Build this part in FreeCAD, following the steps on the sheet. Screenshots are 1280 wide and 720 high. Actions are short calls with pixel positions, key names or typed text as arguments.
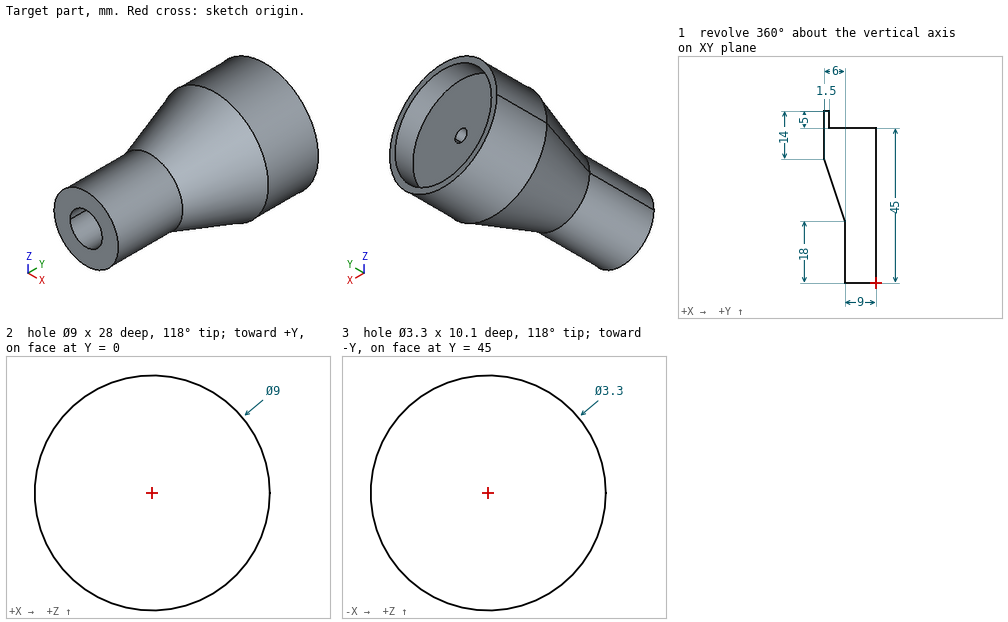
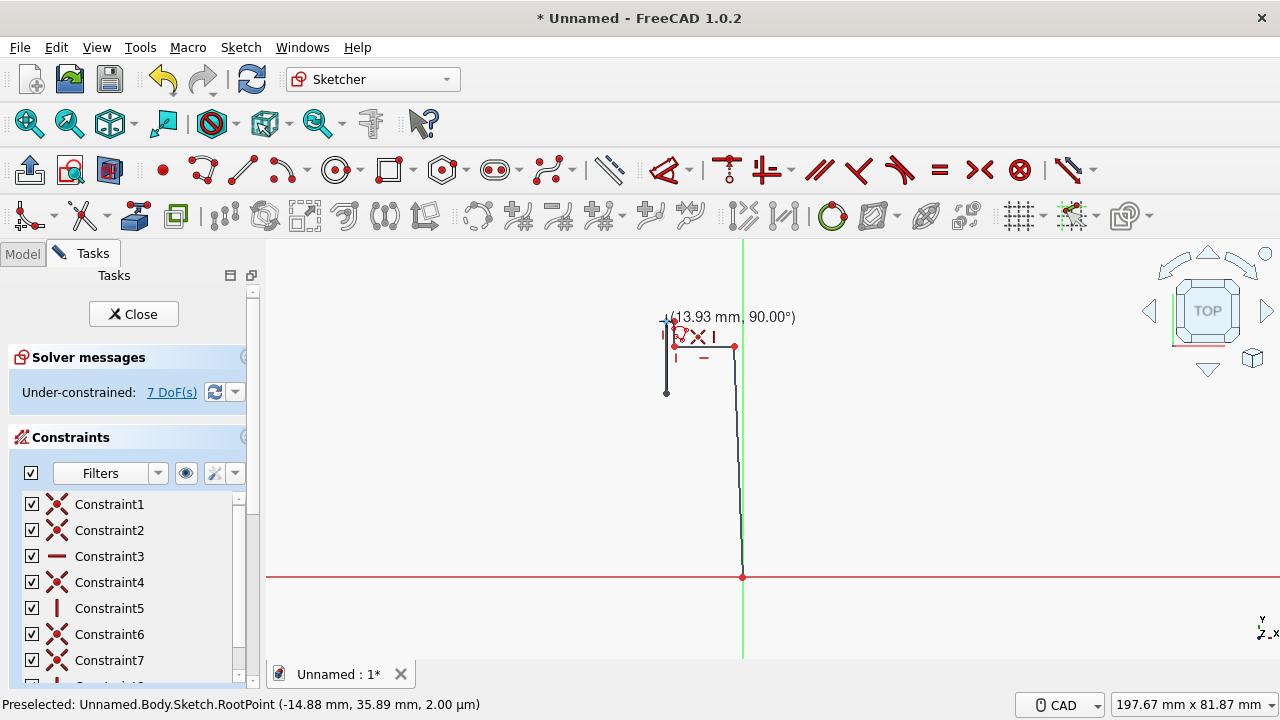
click(697, 485)
click(697, 568)
click(743, 577)
key(Escape)
key(Escape)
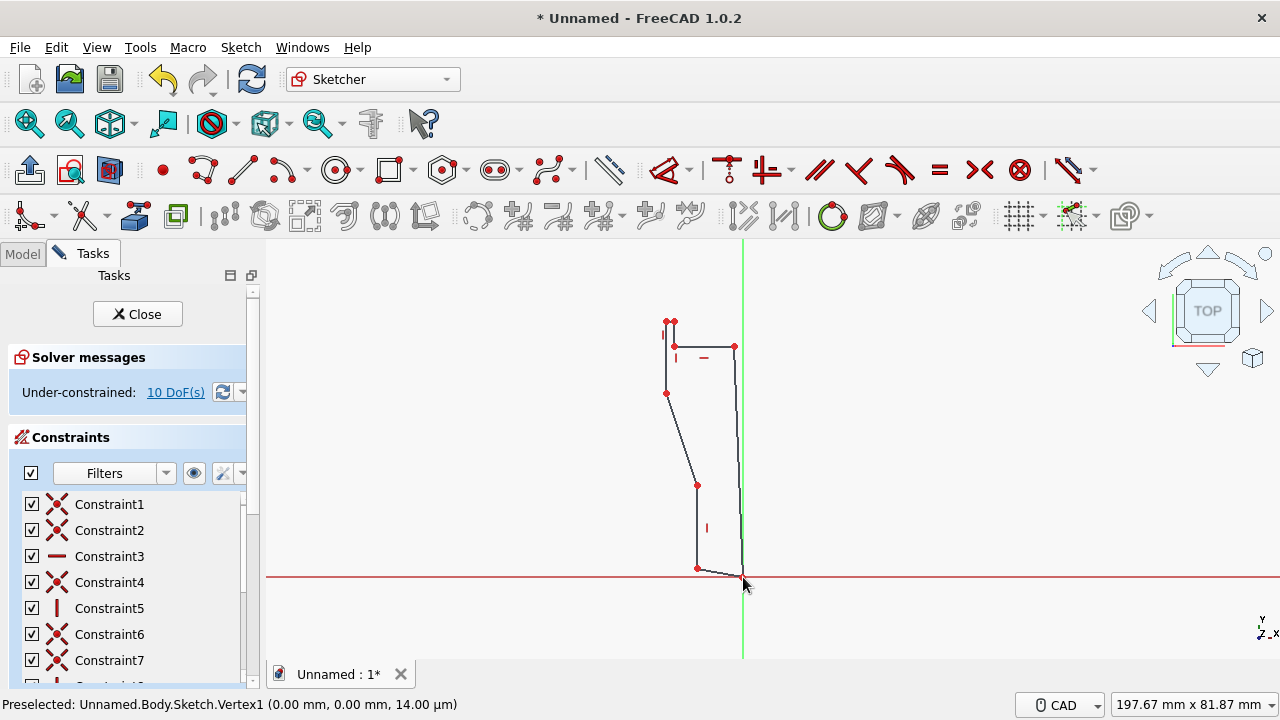
click(740, 508)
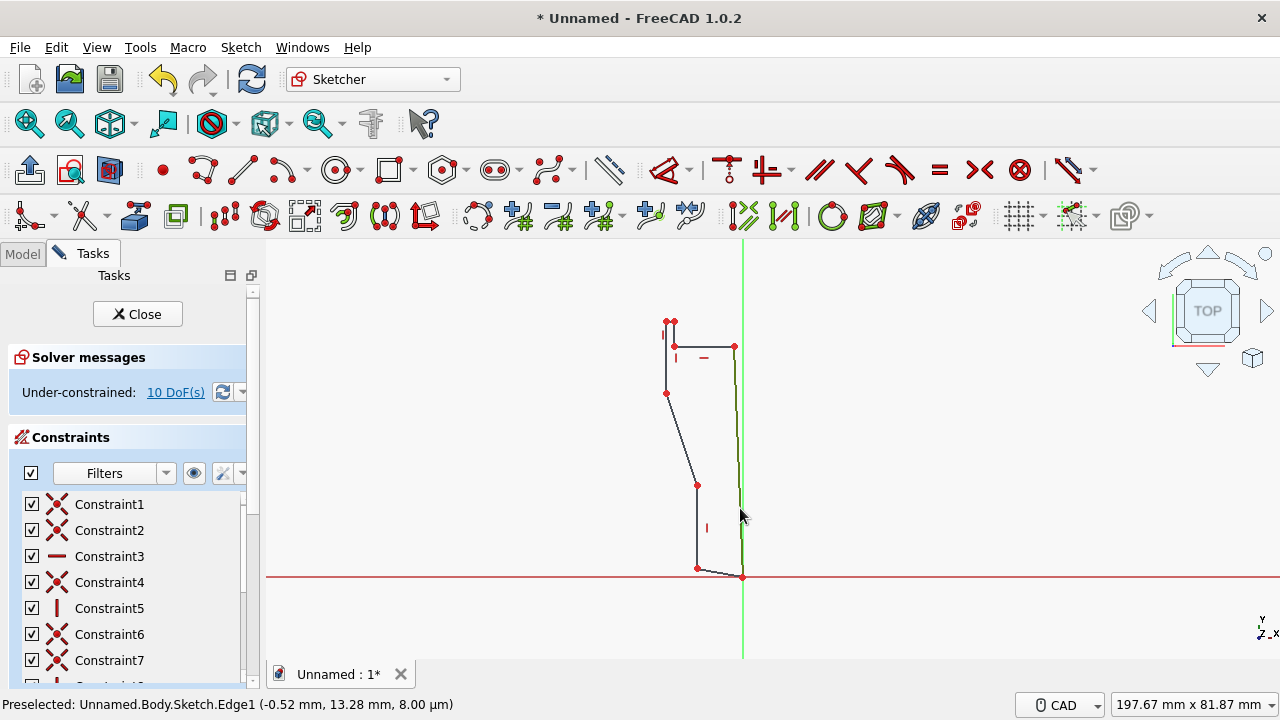
click(794, 170)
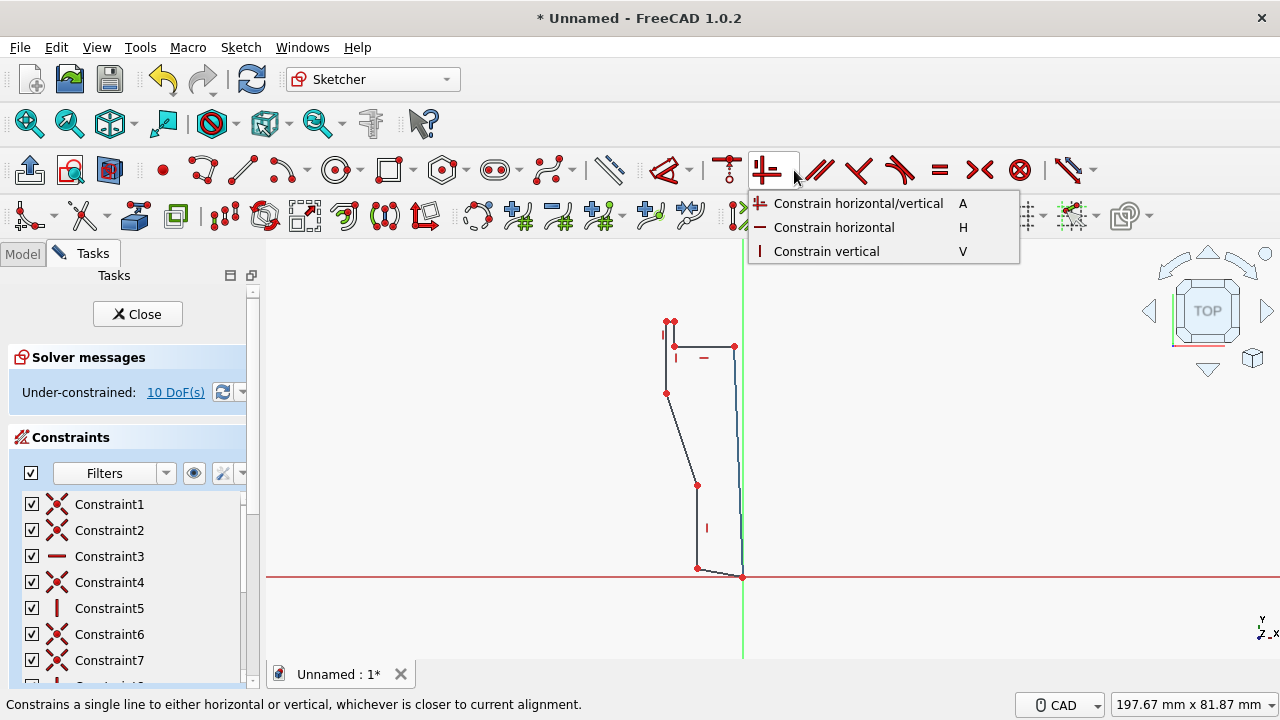
click(884, 251)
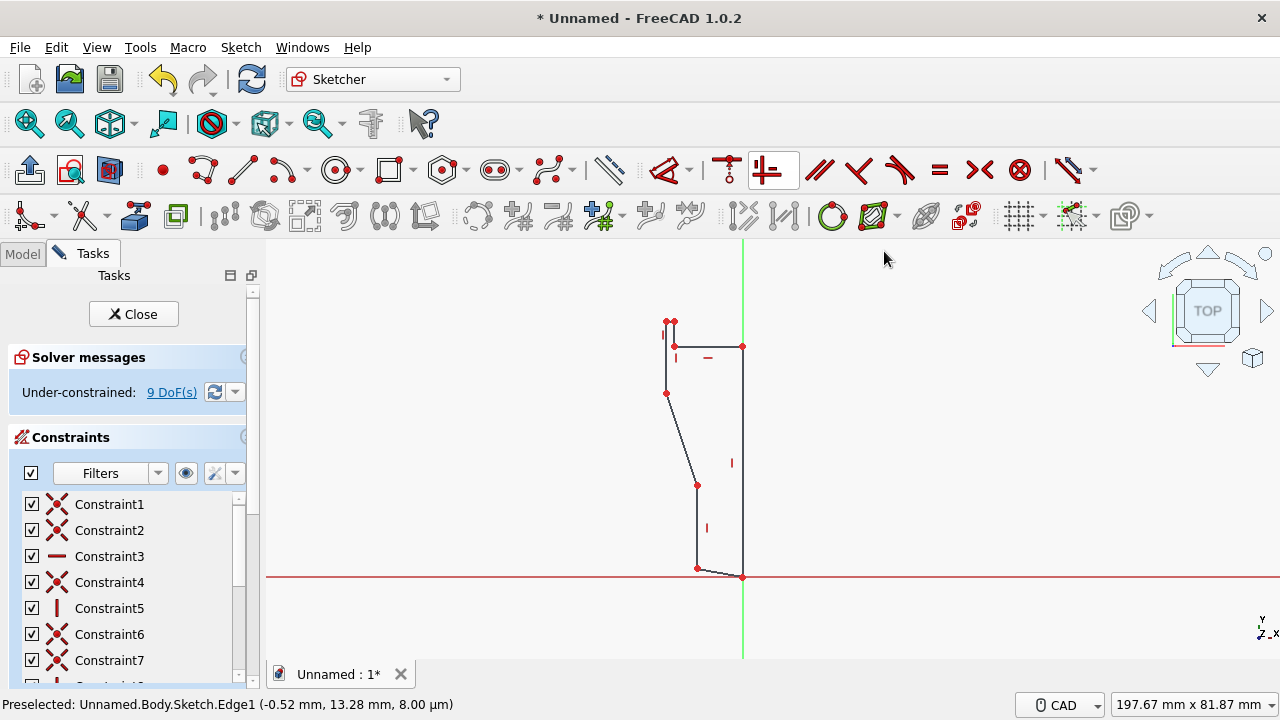
scroll(670, 322, up, 7)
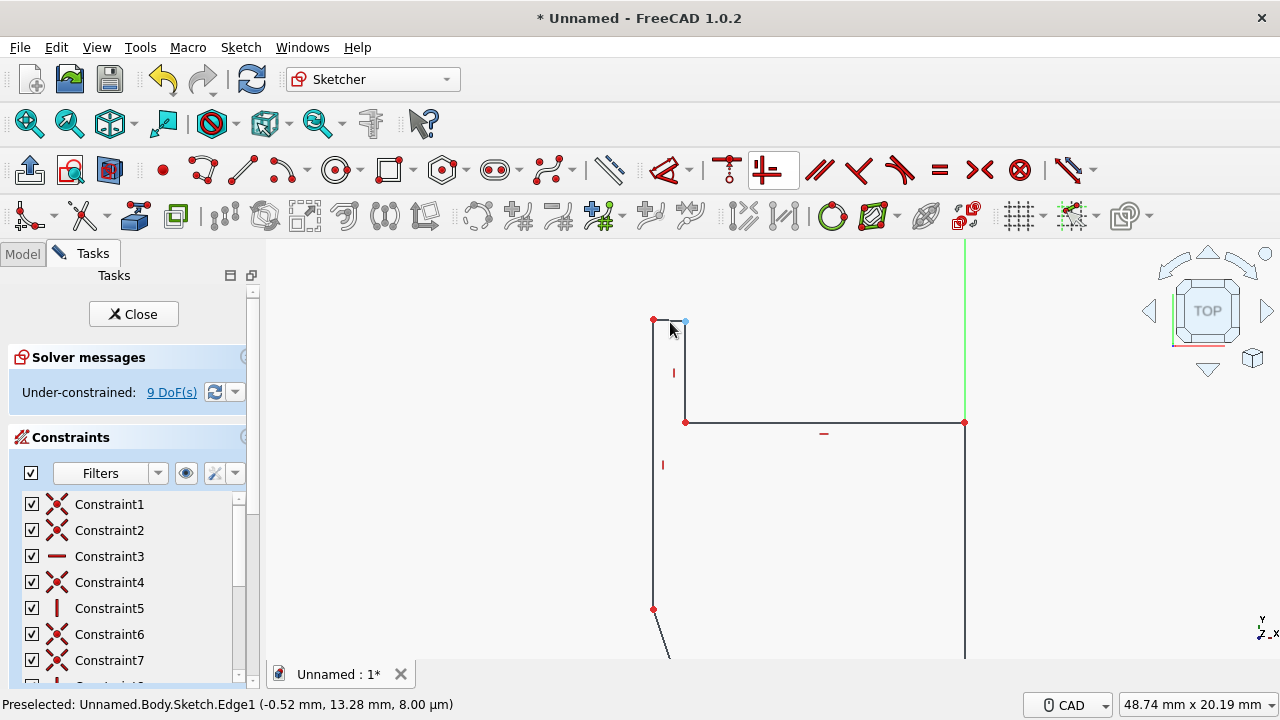
click(669, 320)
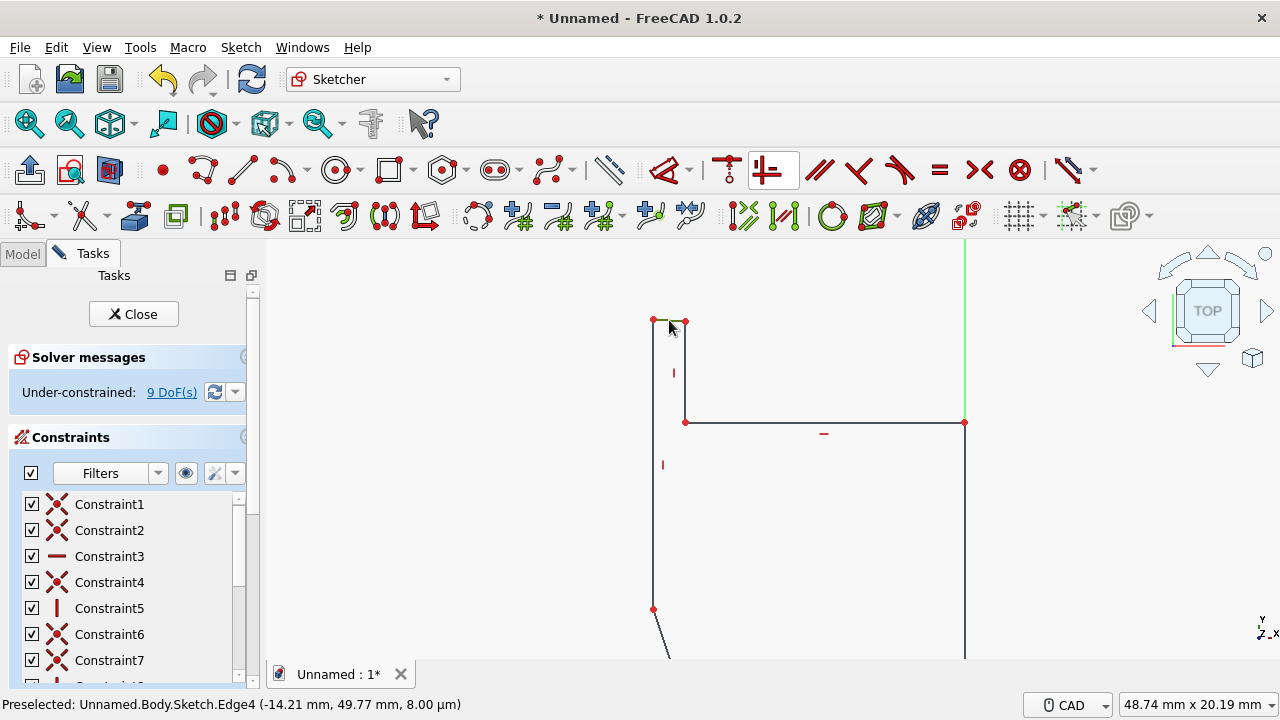
click(794, 170)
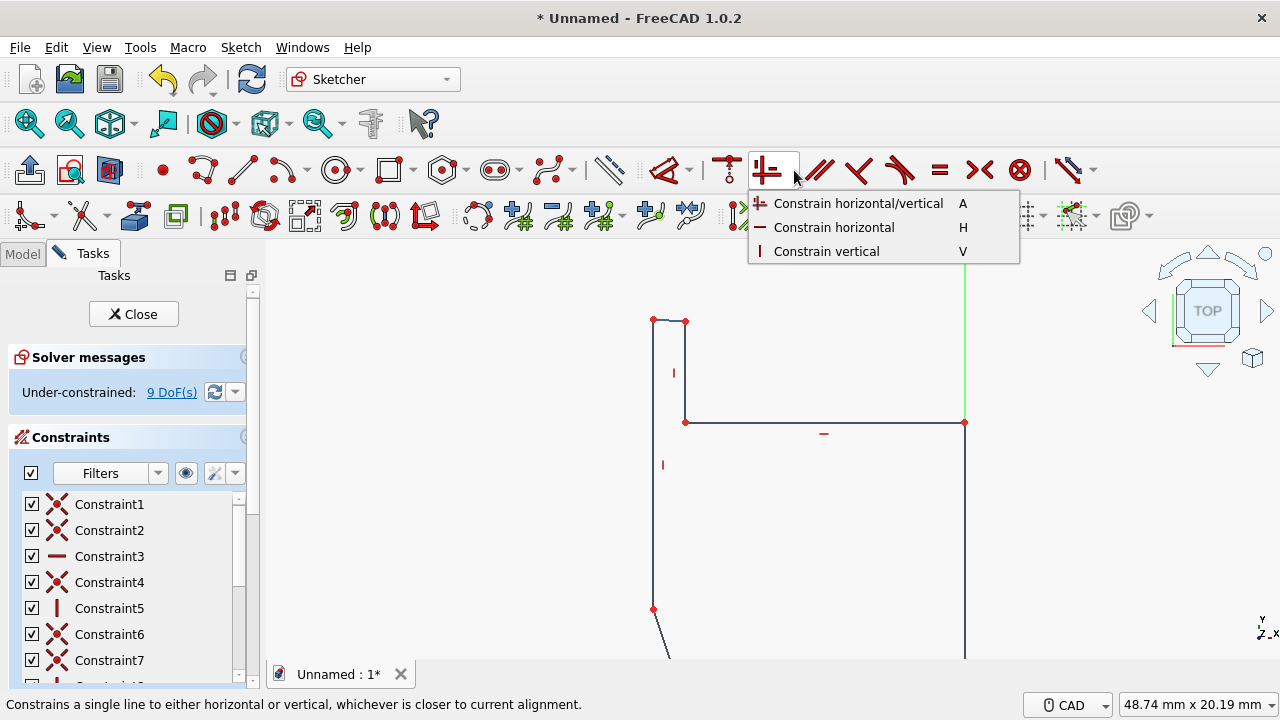
click(884, 227)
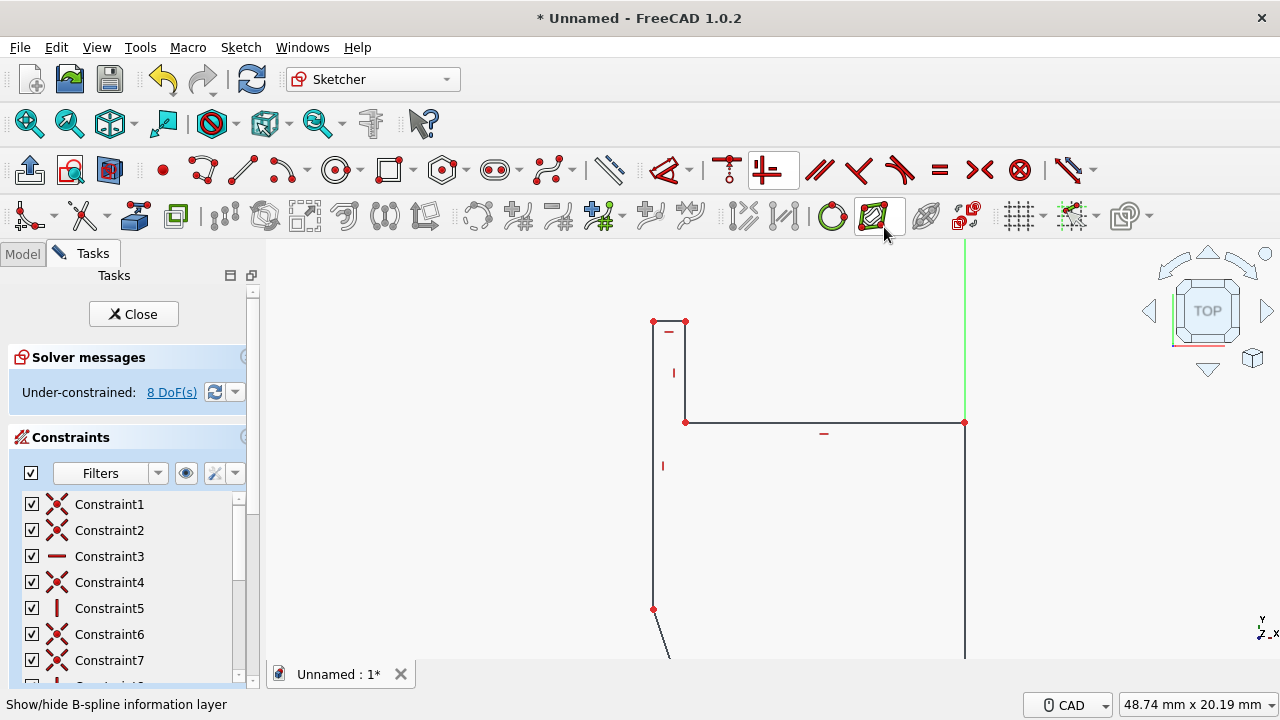
scroll(670, 322, down, 7)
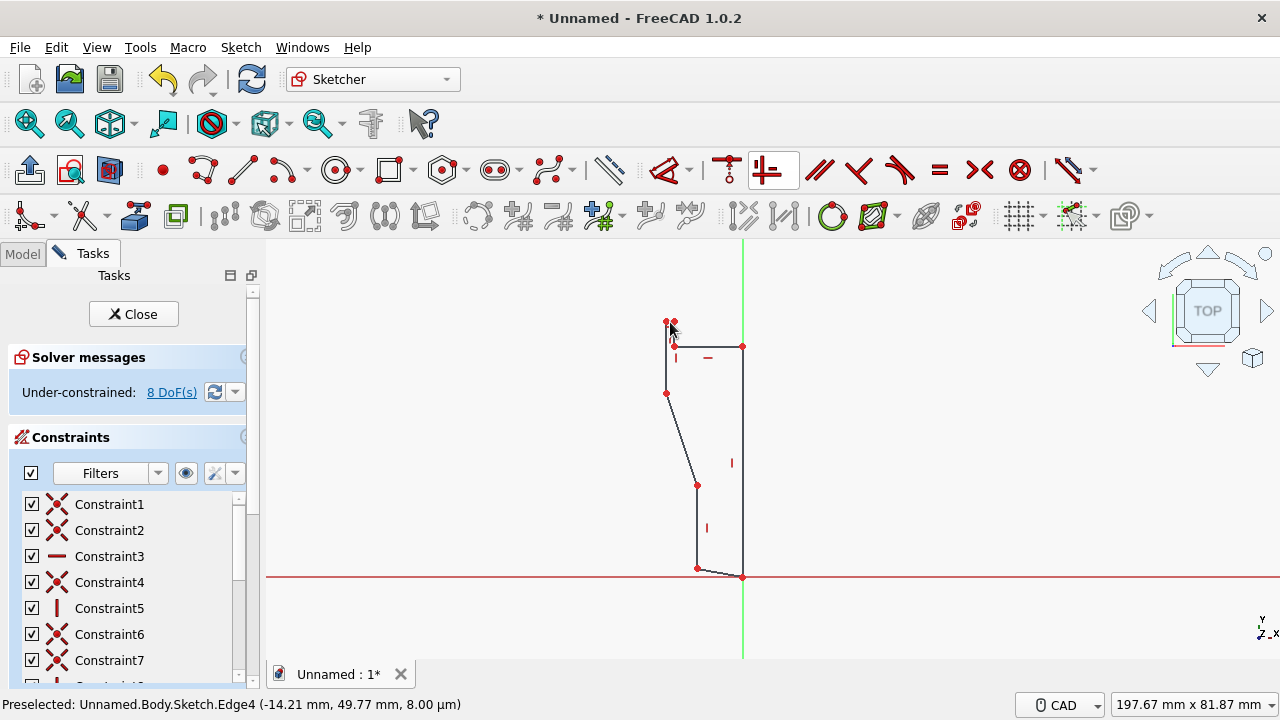
scroll(711, 571, up, 5)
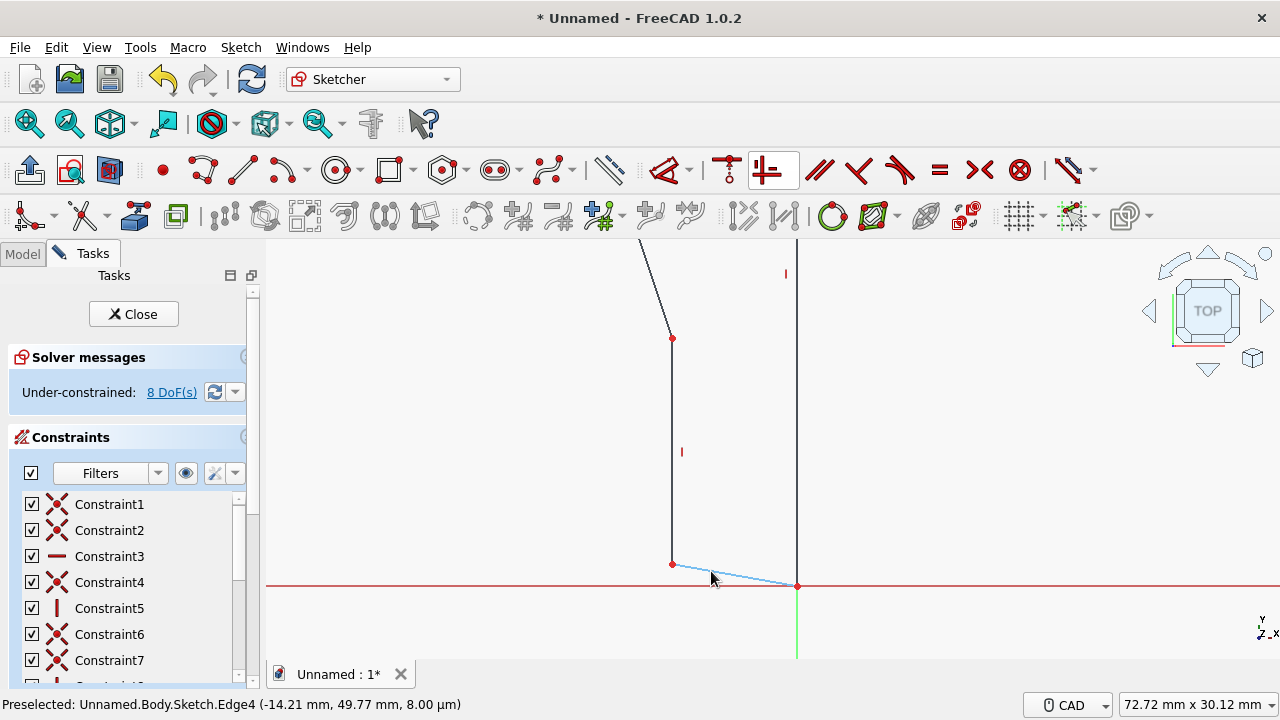
click(710, 571)